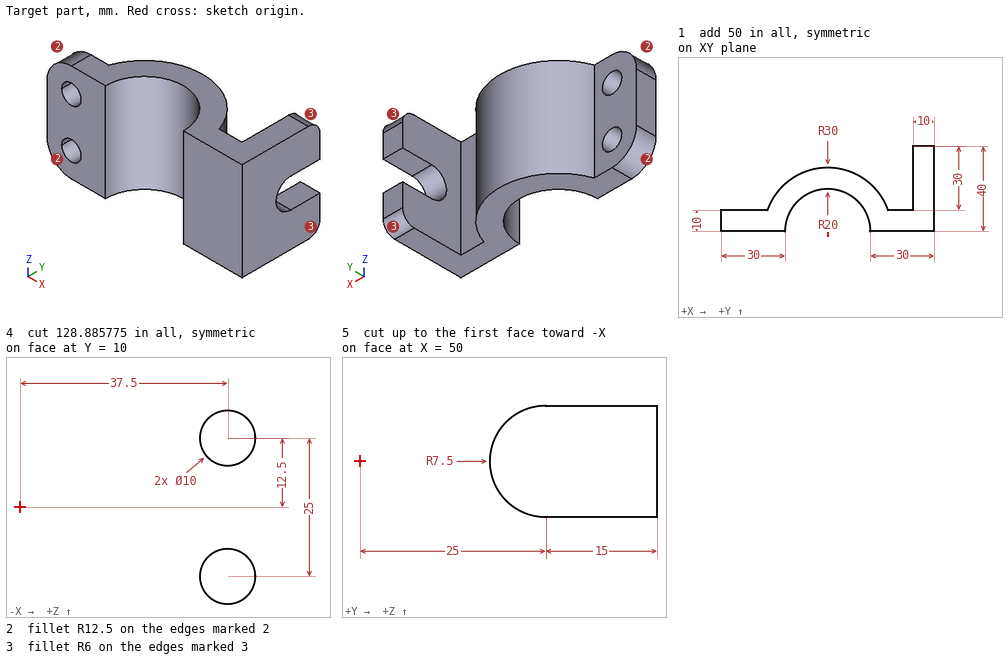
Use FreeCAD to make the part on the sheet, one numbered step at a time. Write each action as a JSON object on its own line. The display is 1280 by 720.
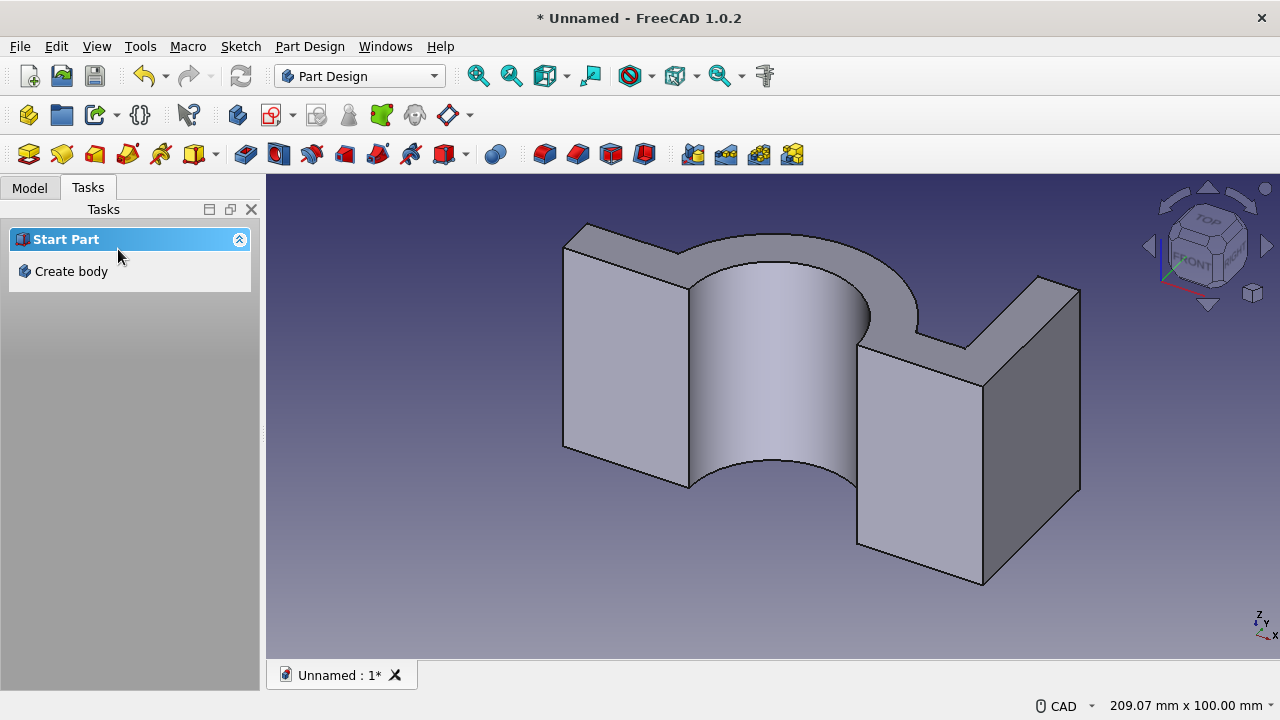
{"action": "left_click", "coordinate": [479, 76]}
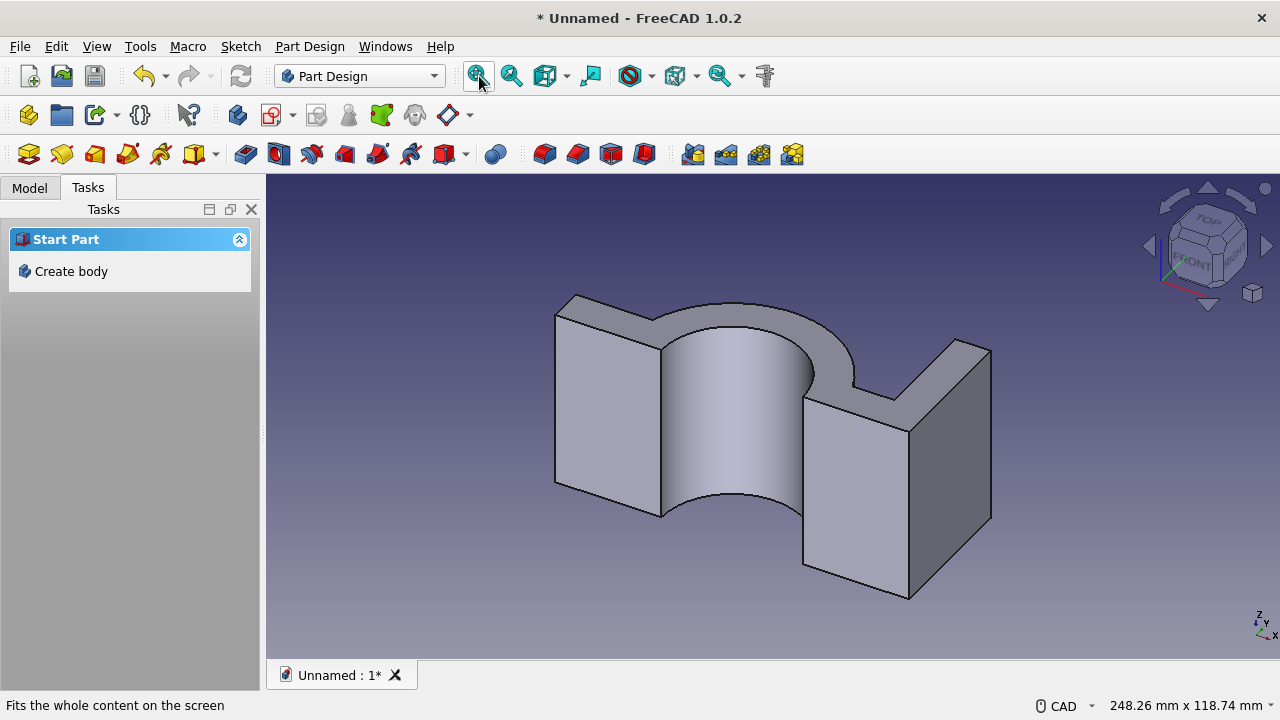
{"action": "key", "text": "0"}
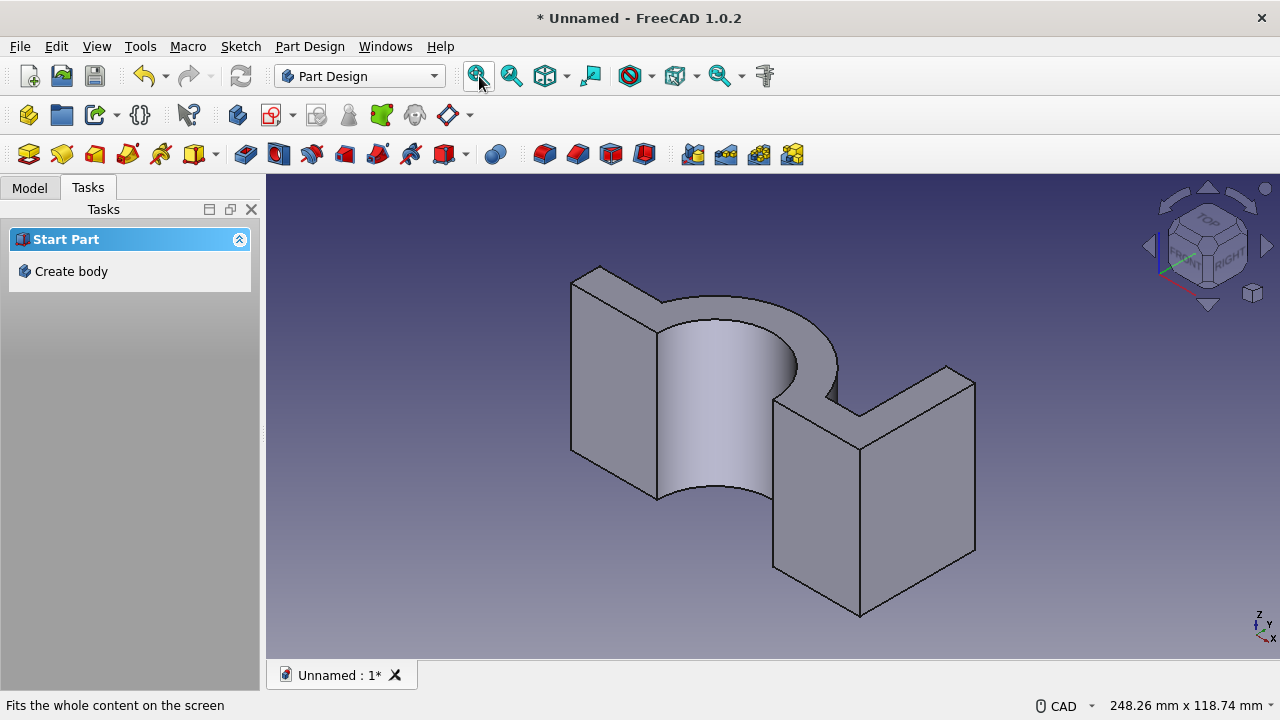
{"action": "key", "text": "2"}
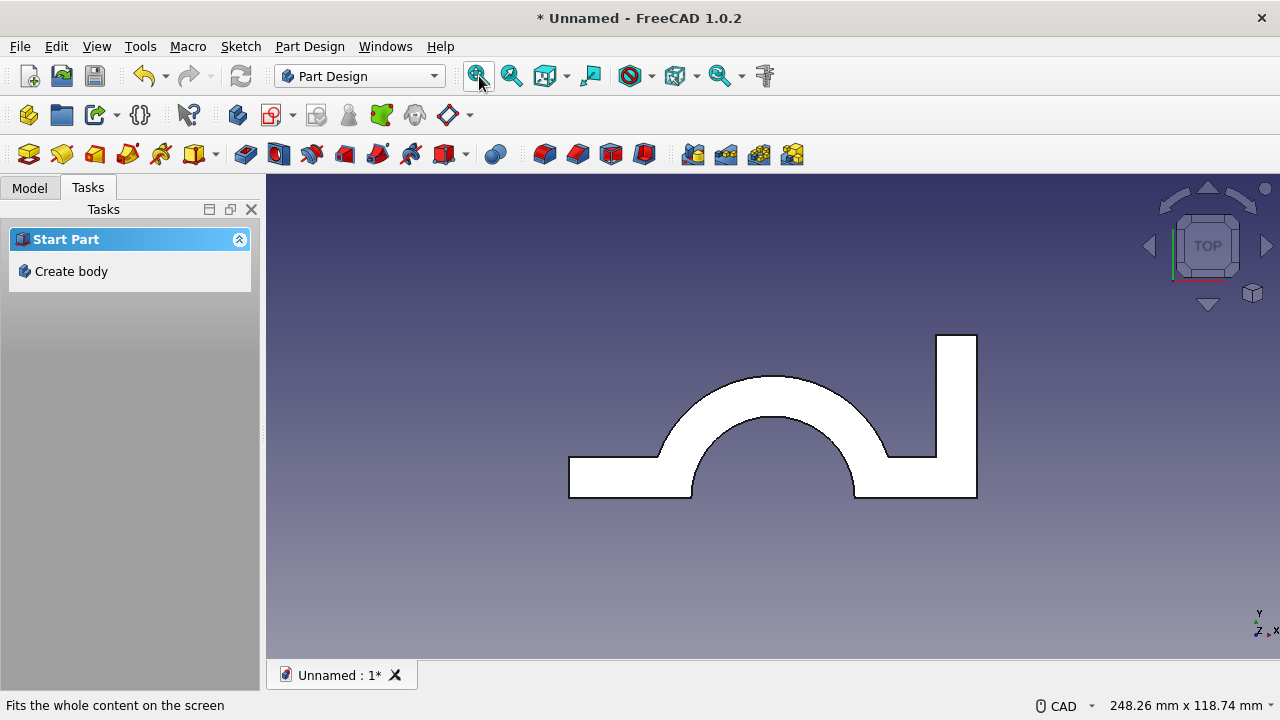
{"action": "left_click", "coordinate": [479, 76]}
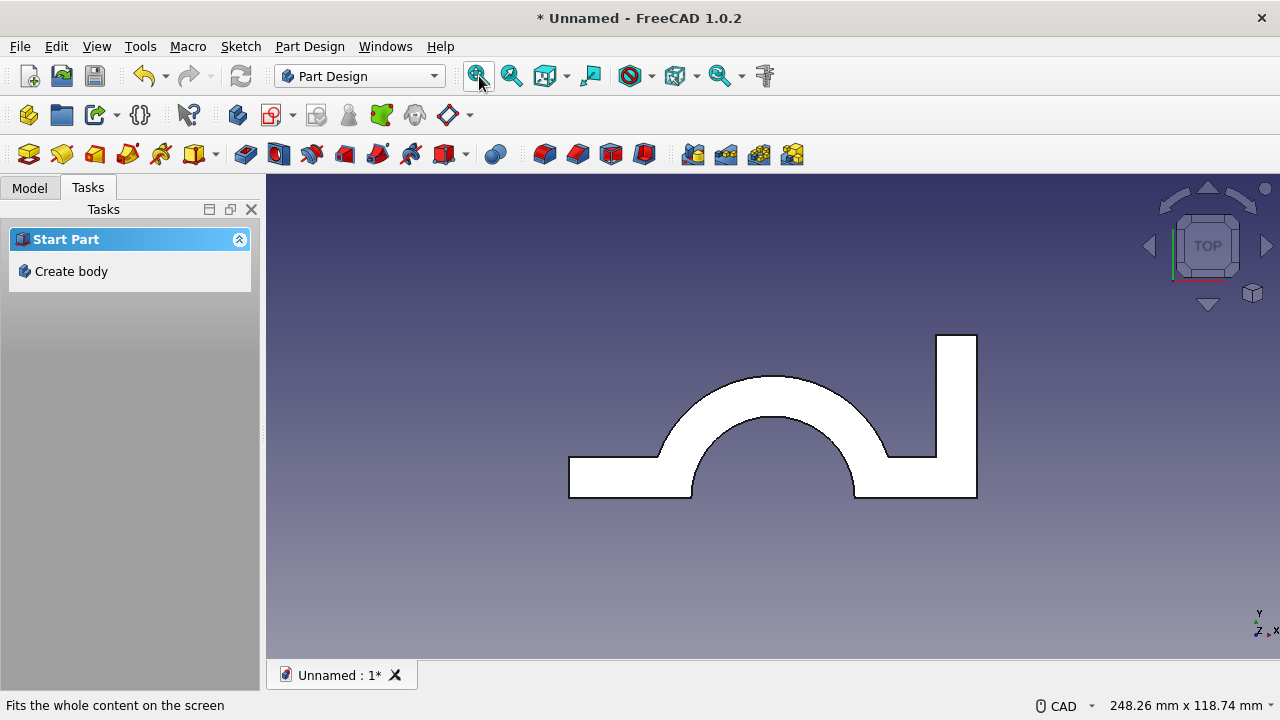
{"action": "left_click", "coordinate": [569, 477]}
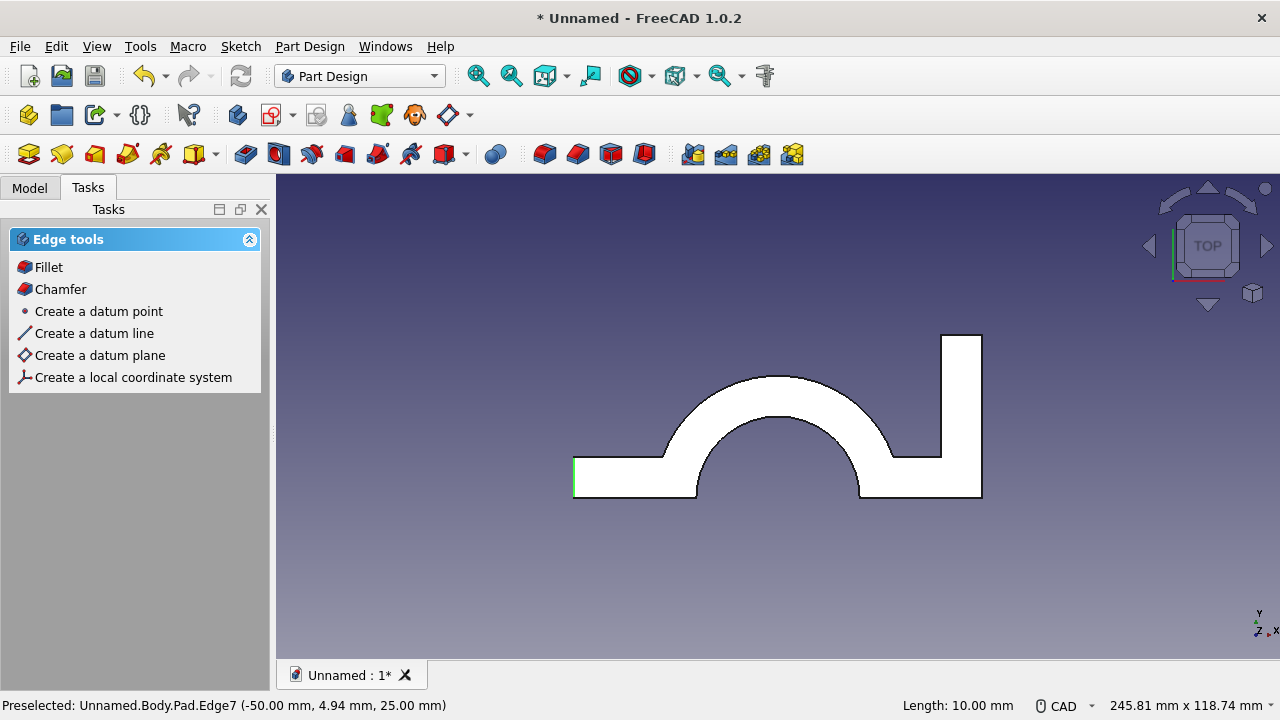
{"action": "key", "text": "1"}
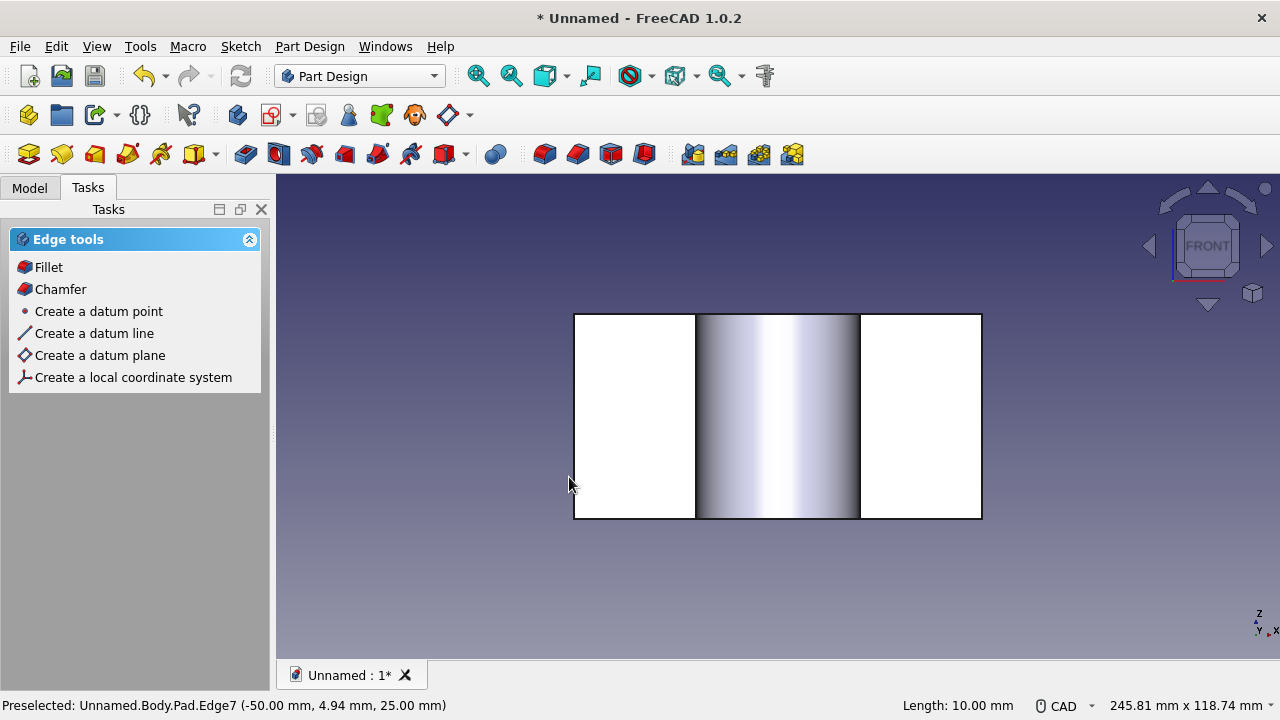
{"action": "left_click", "coordinate": [479, 76]}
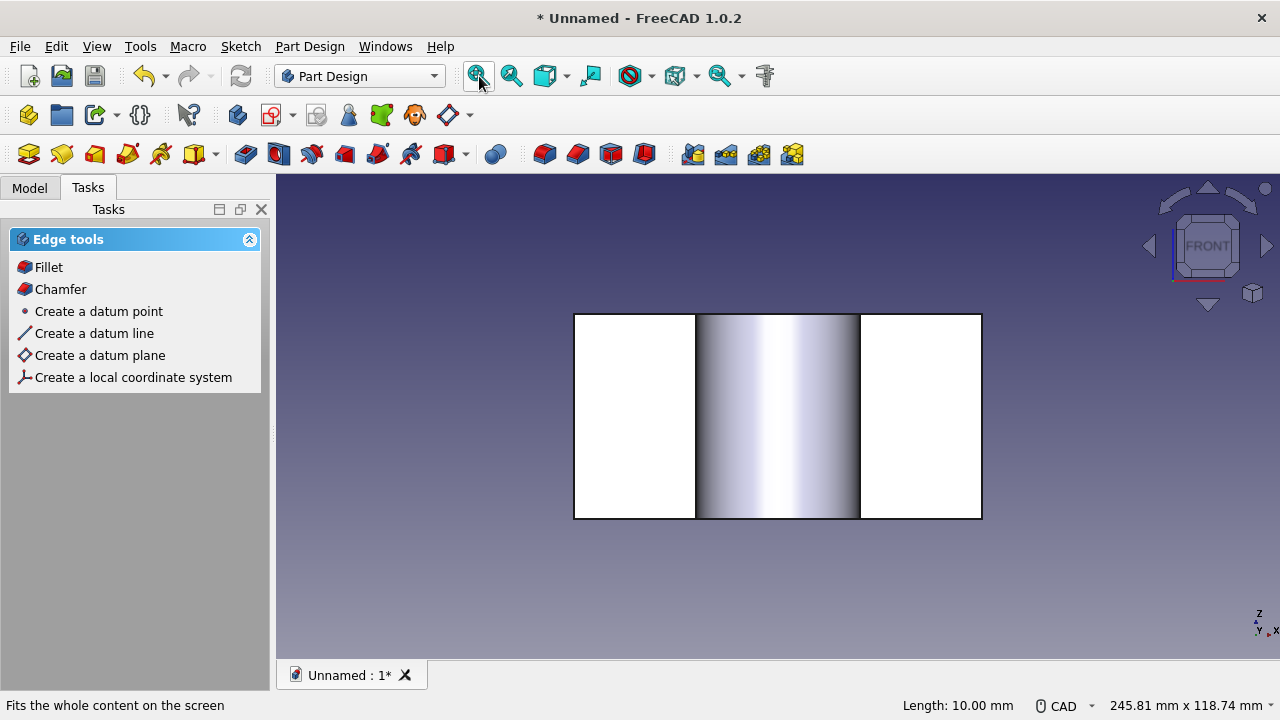
{"action": "key", "text": "3"}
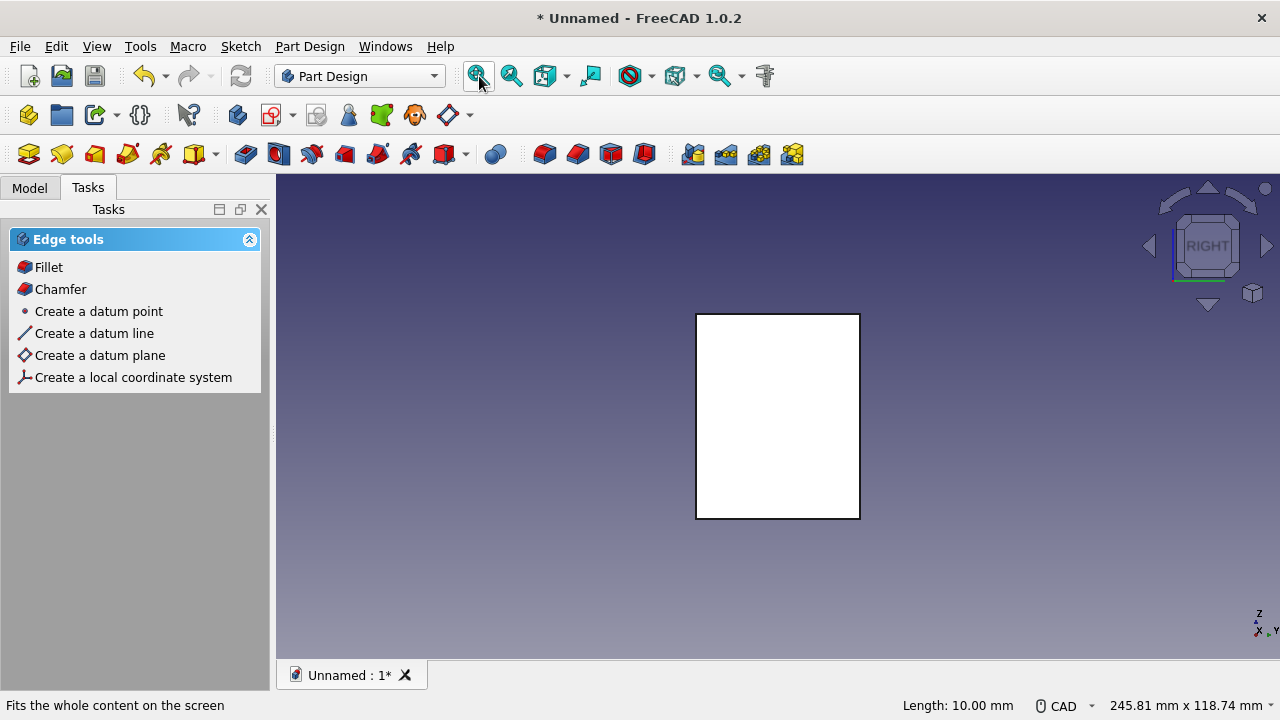
{"action": "left_click", "coordinate": [479, 76]}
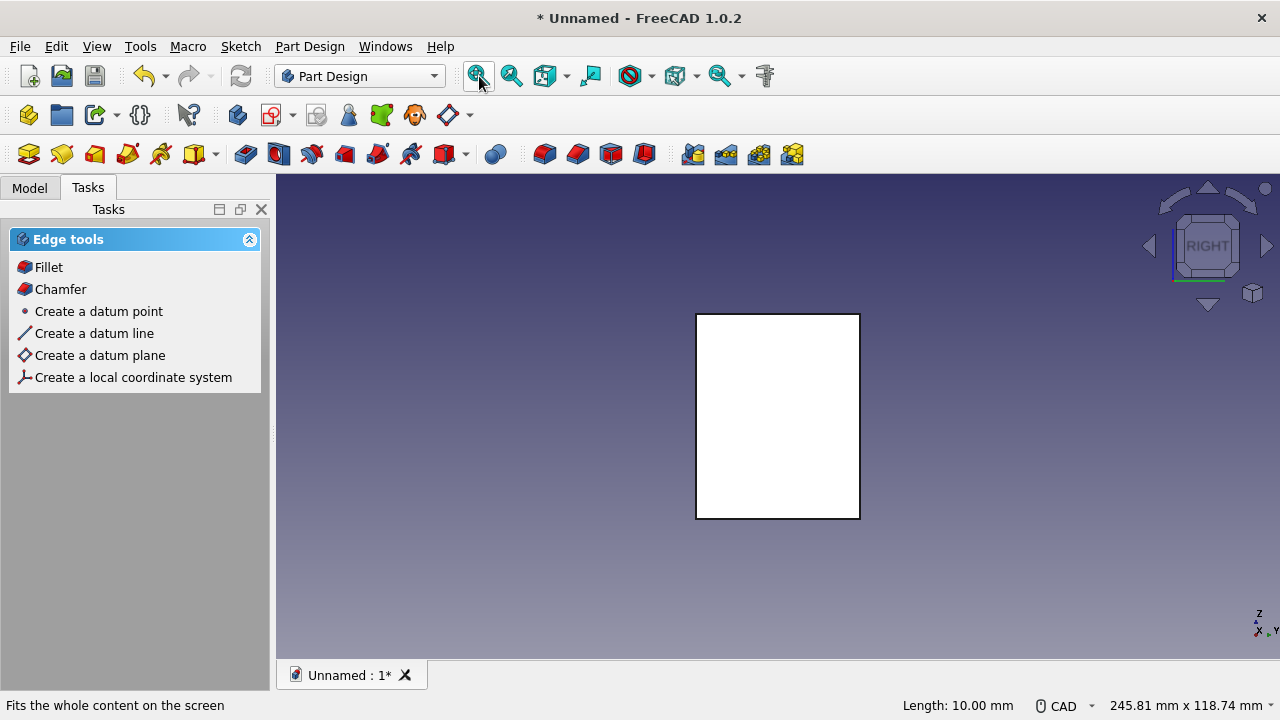
{"action": "key", "text": "5"}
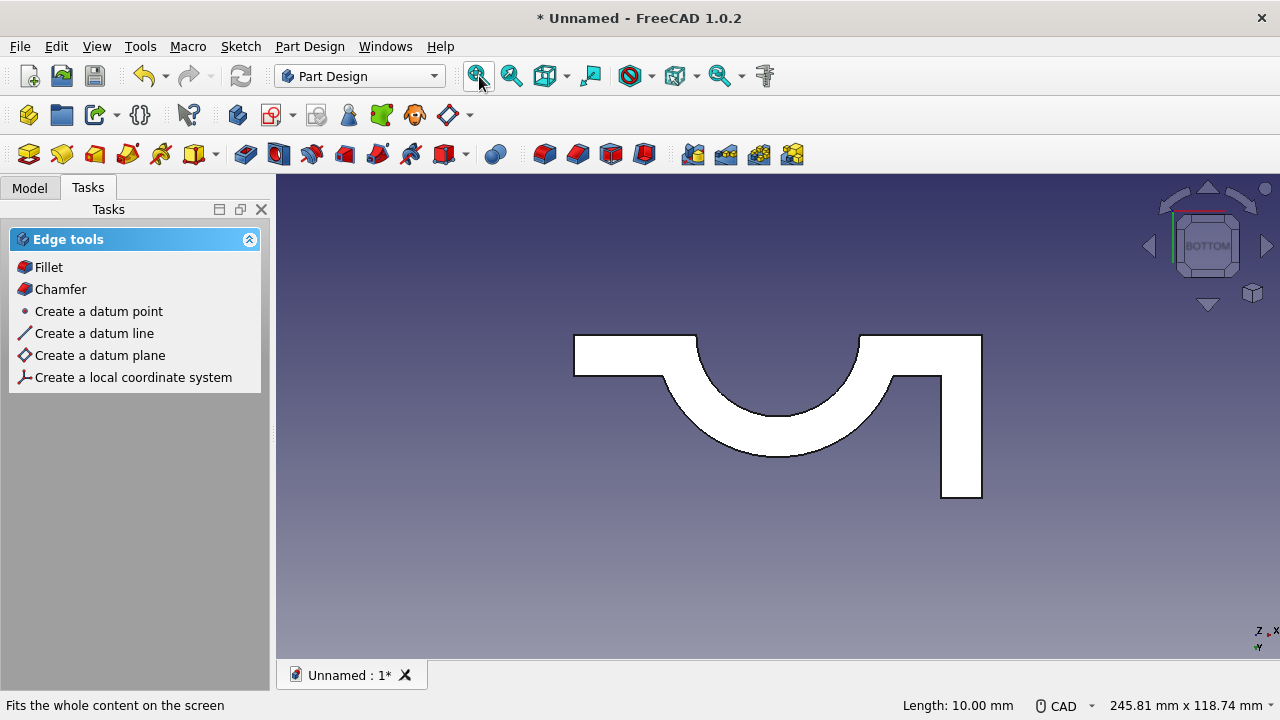
{"action": "left_click", "coordinate": [479, 76]}